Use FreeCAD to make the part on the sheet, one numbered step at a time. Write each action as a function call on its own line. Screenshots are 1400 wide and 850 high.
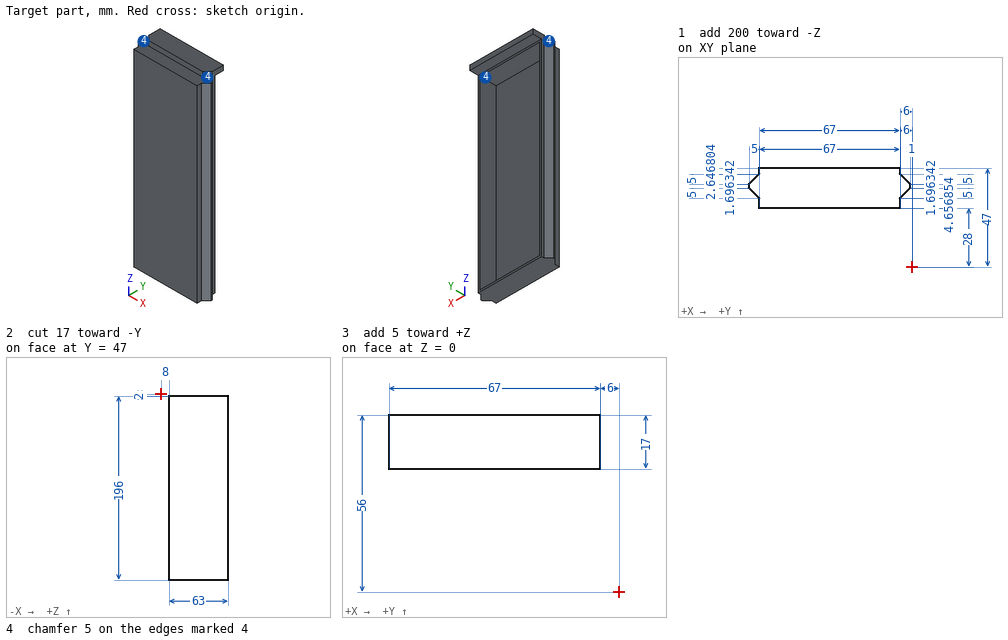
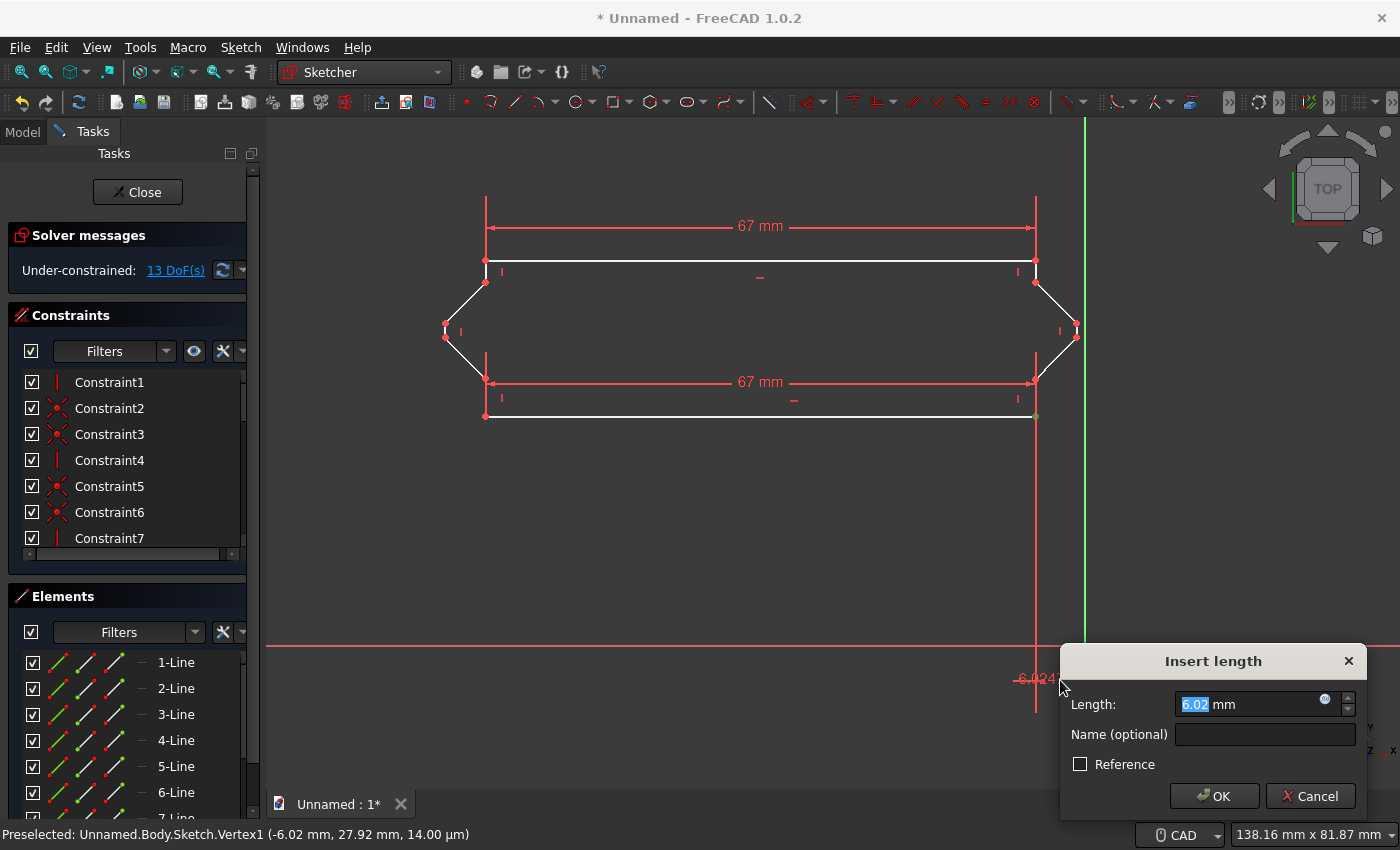
text(6)
key(Return)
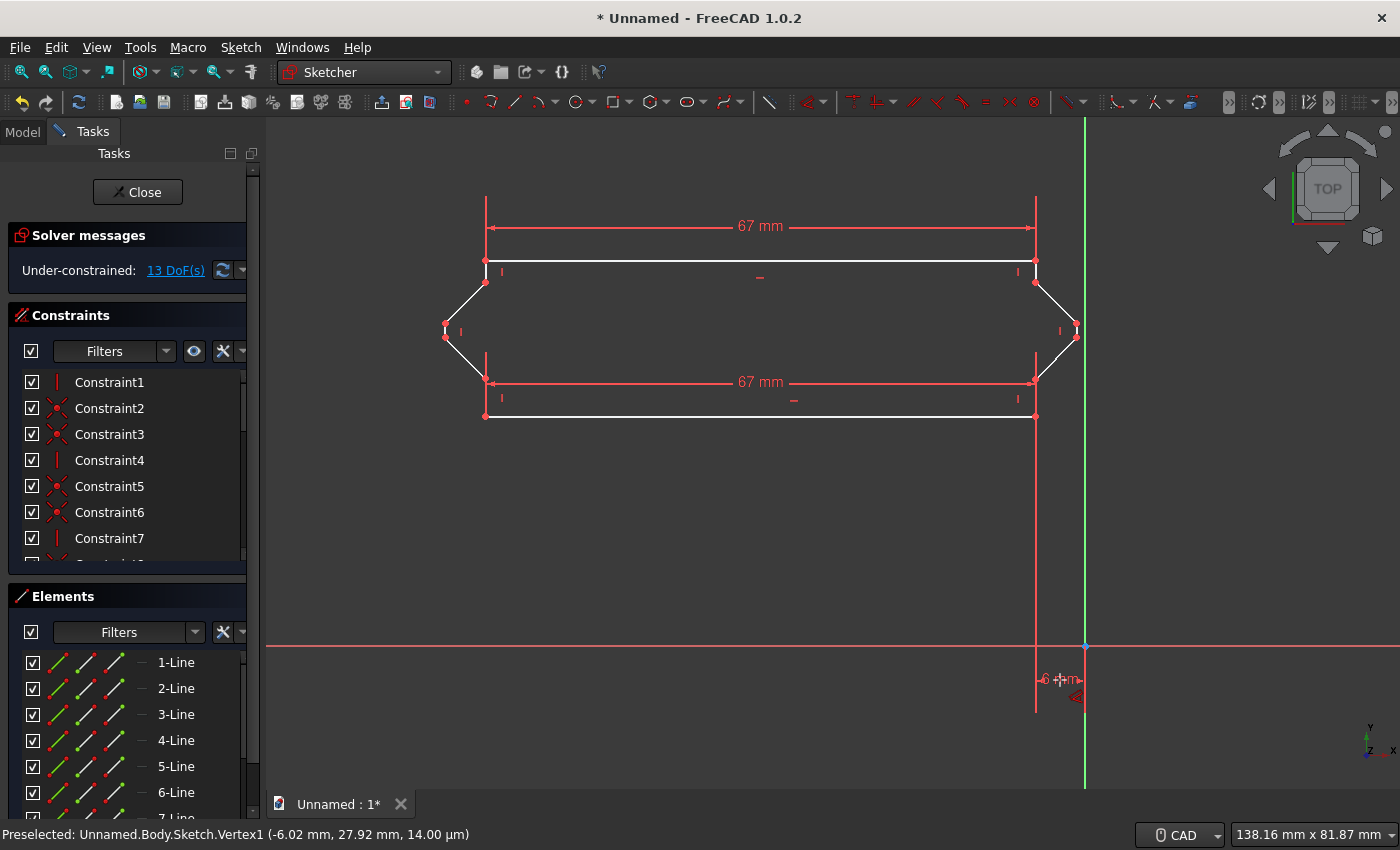
scroll(1077, 338, up, 8)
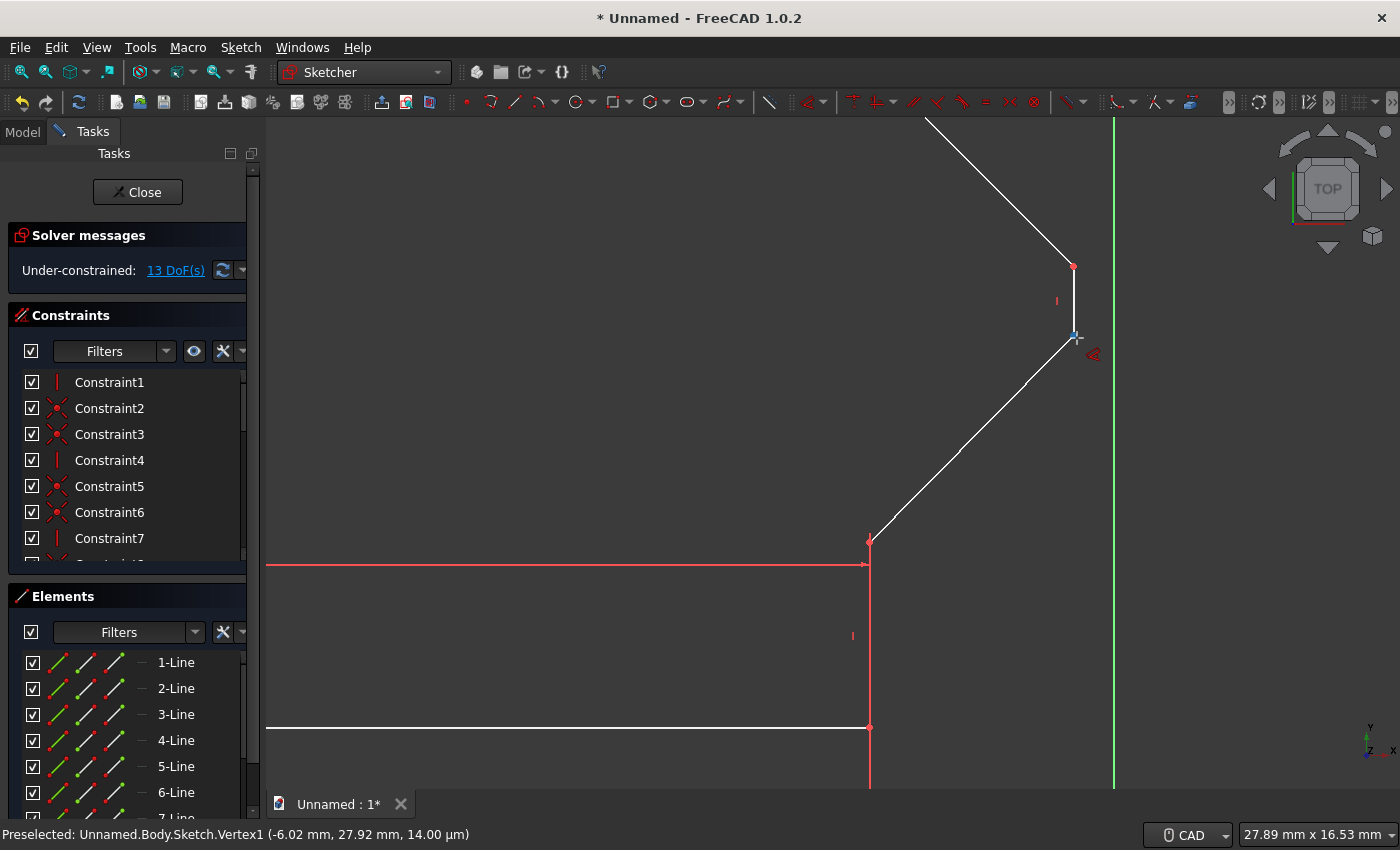
click(1074, 335)
click(1094, 301)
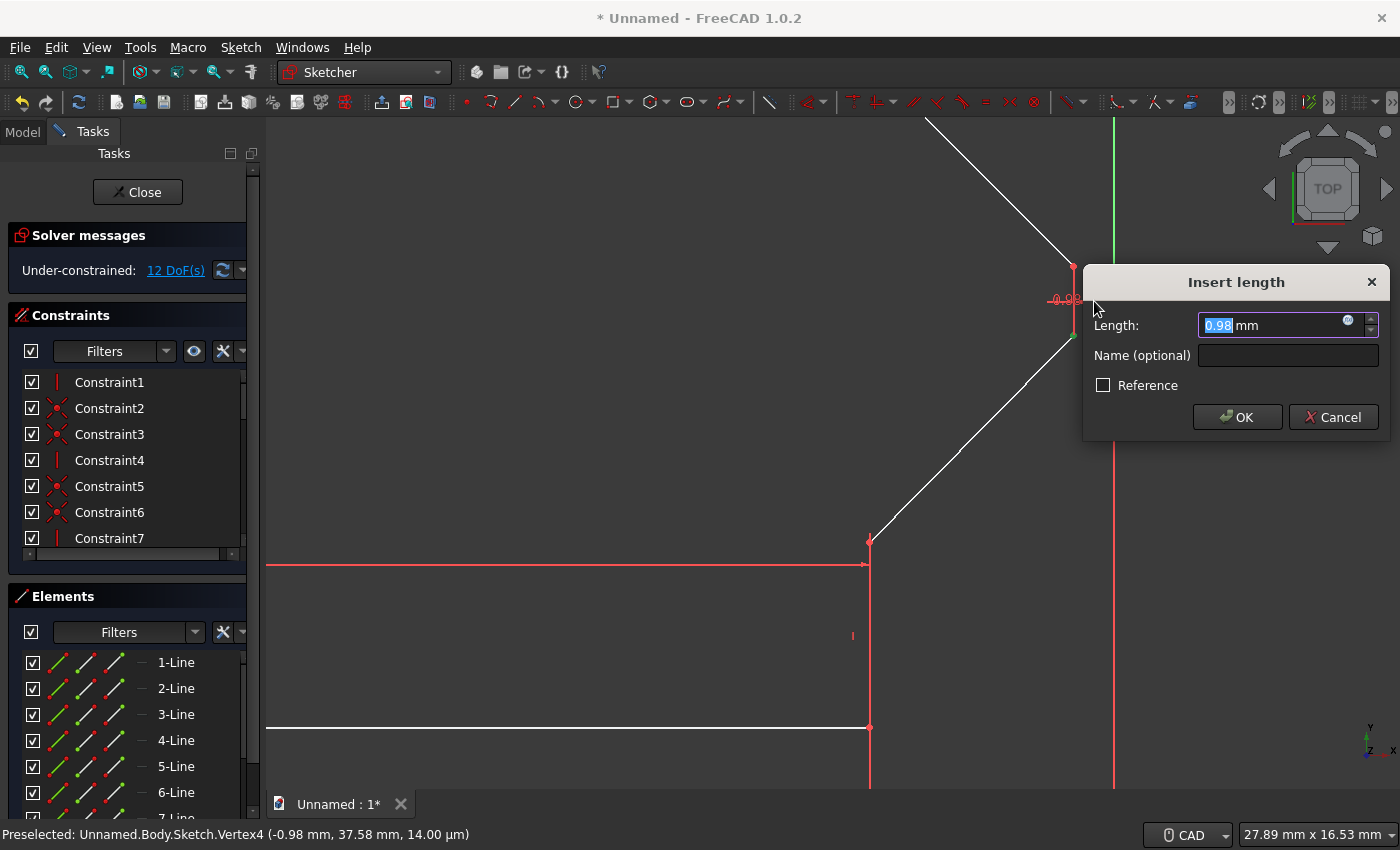
text(1)
key(Return)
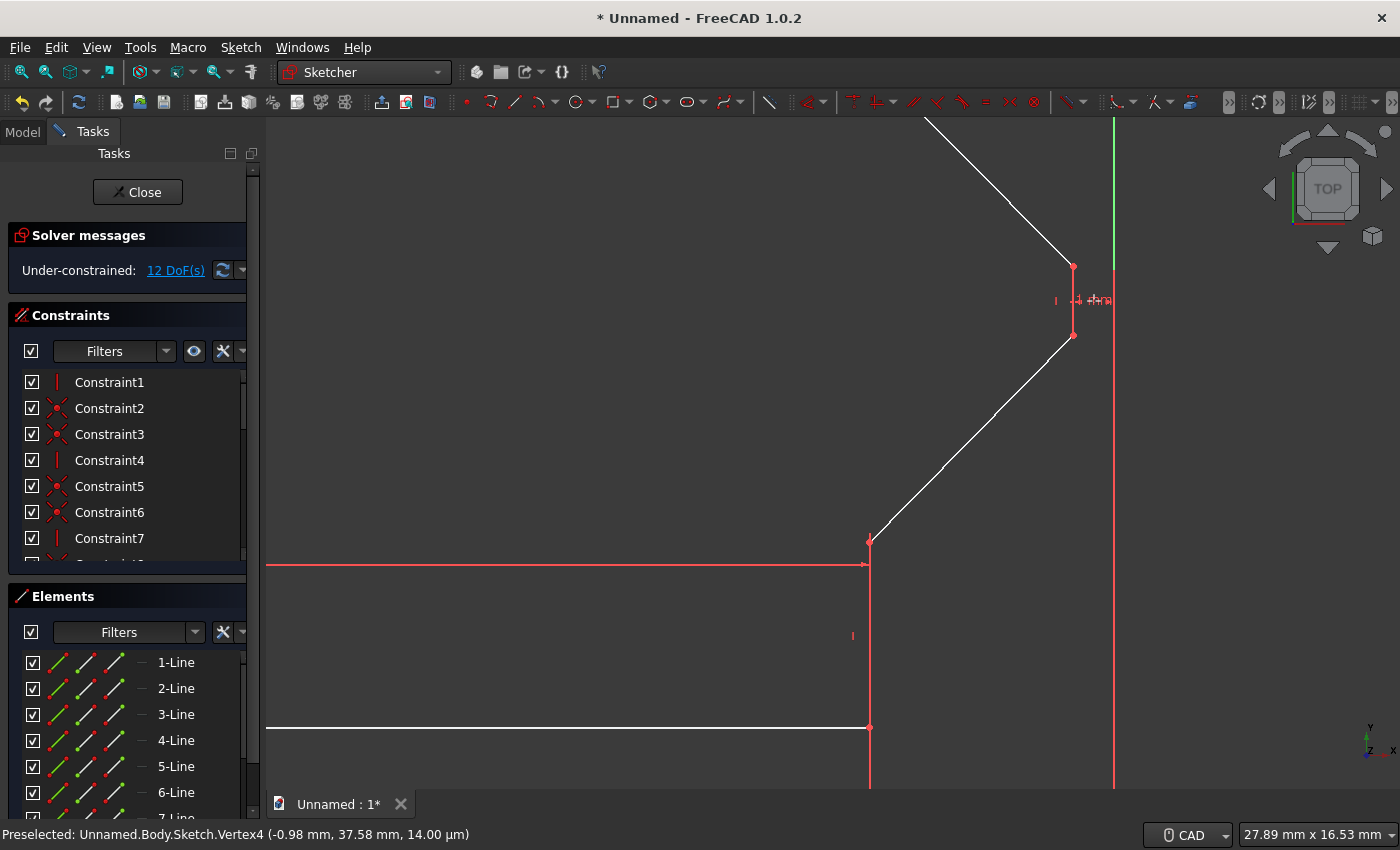
scroll(1077, 338, down, 8)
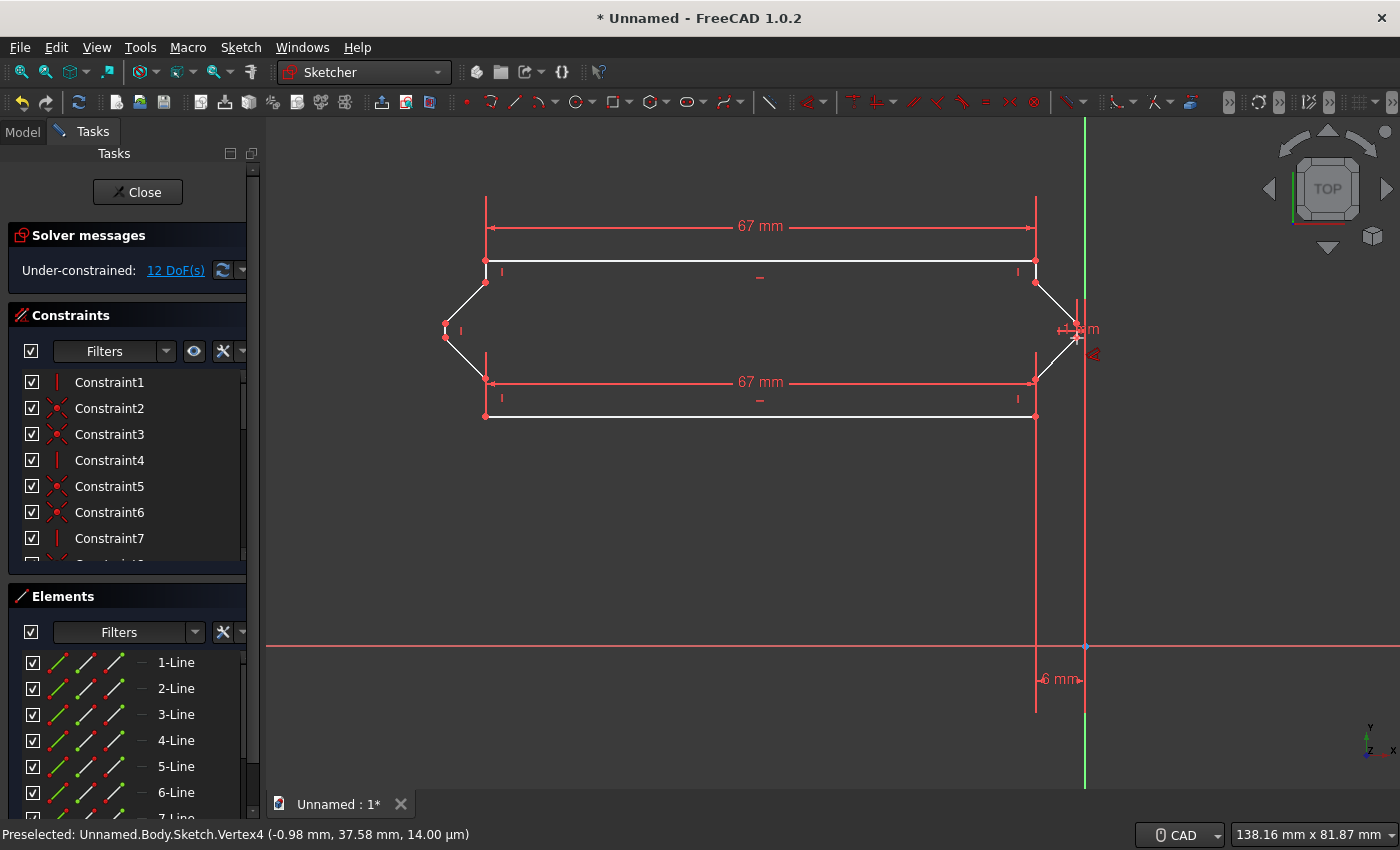
click(1036, 282)
click(1060, 248)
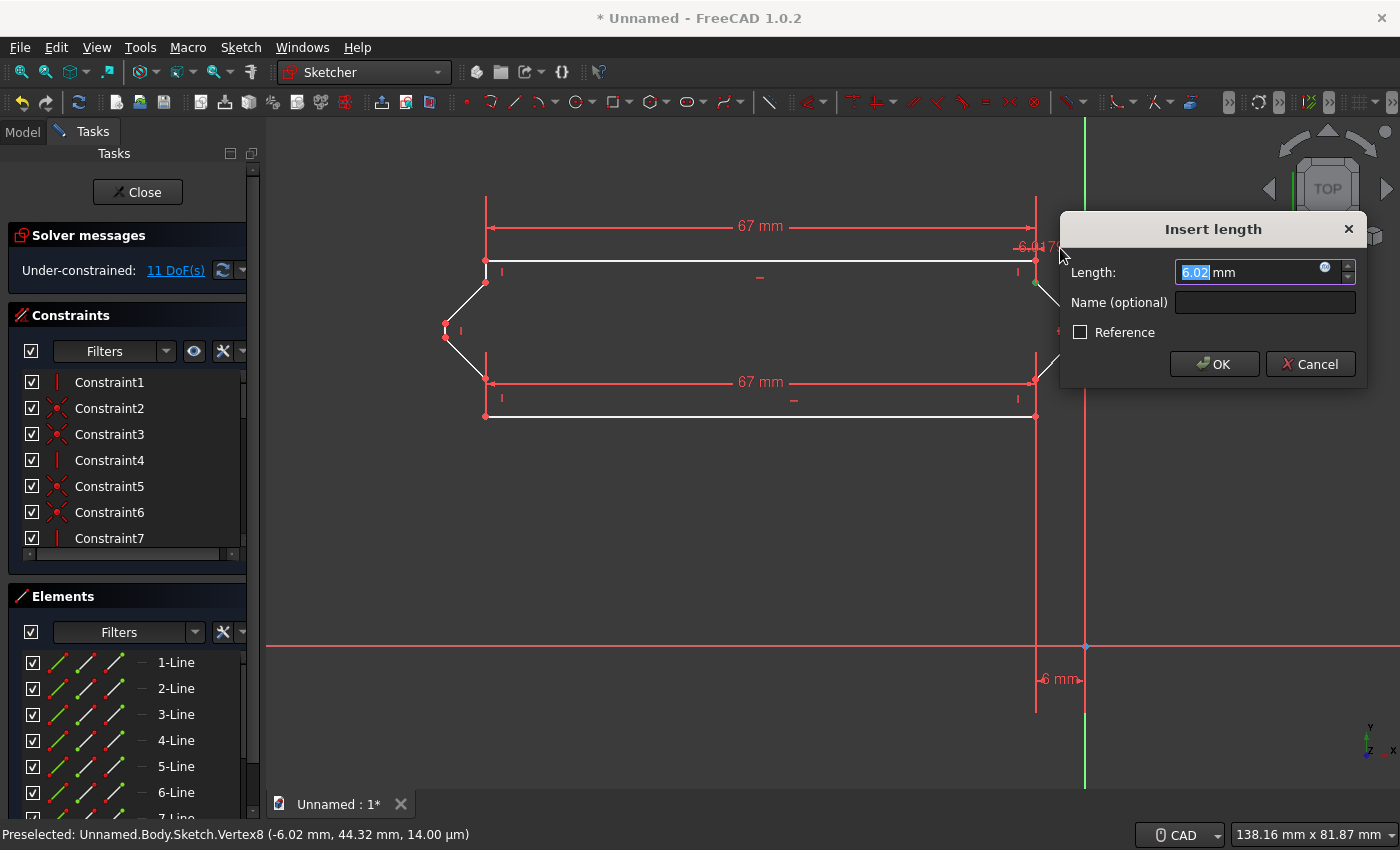
text(6)
key(Return)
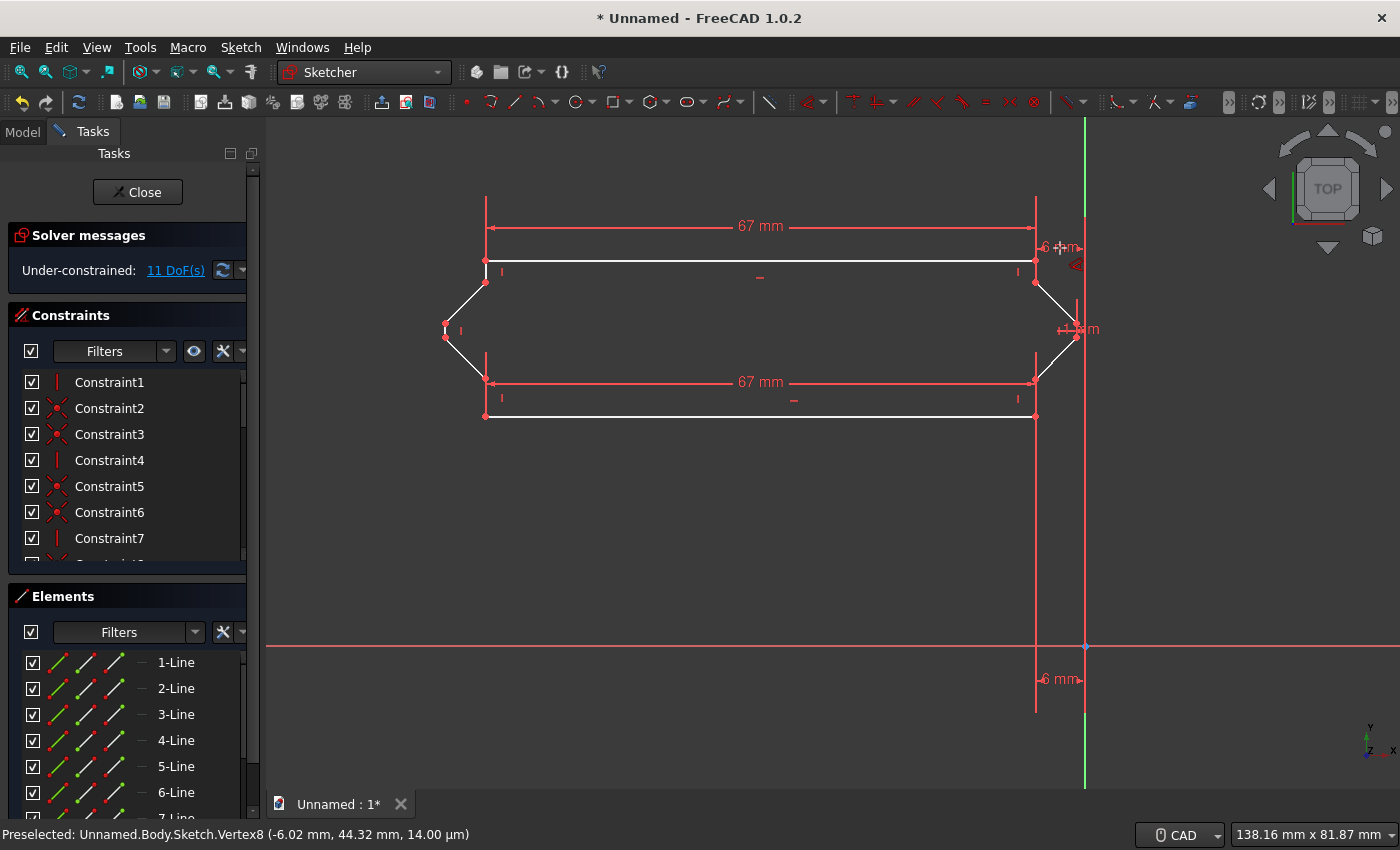
click(1048, 367)
click(1111, 359)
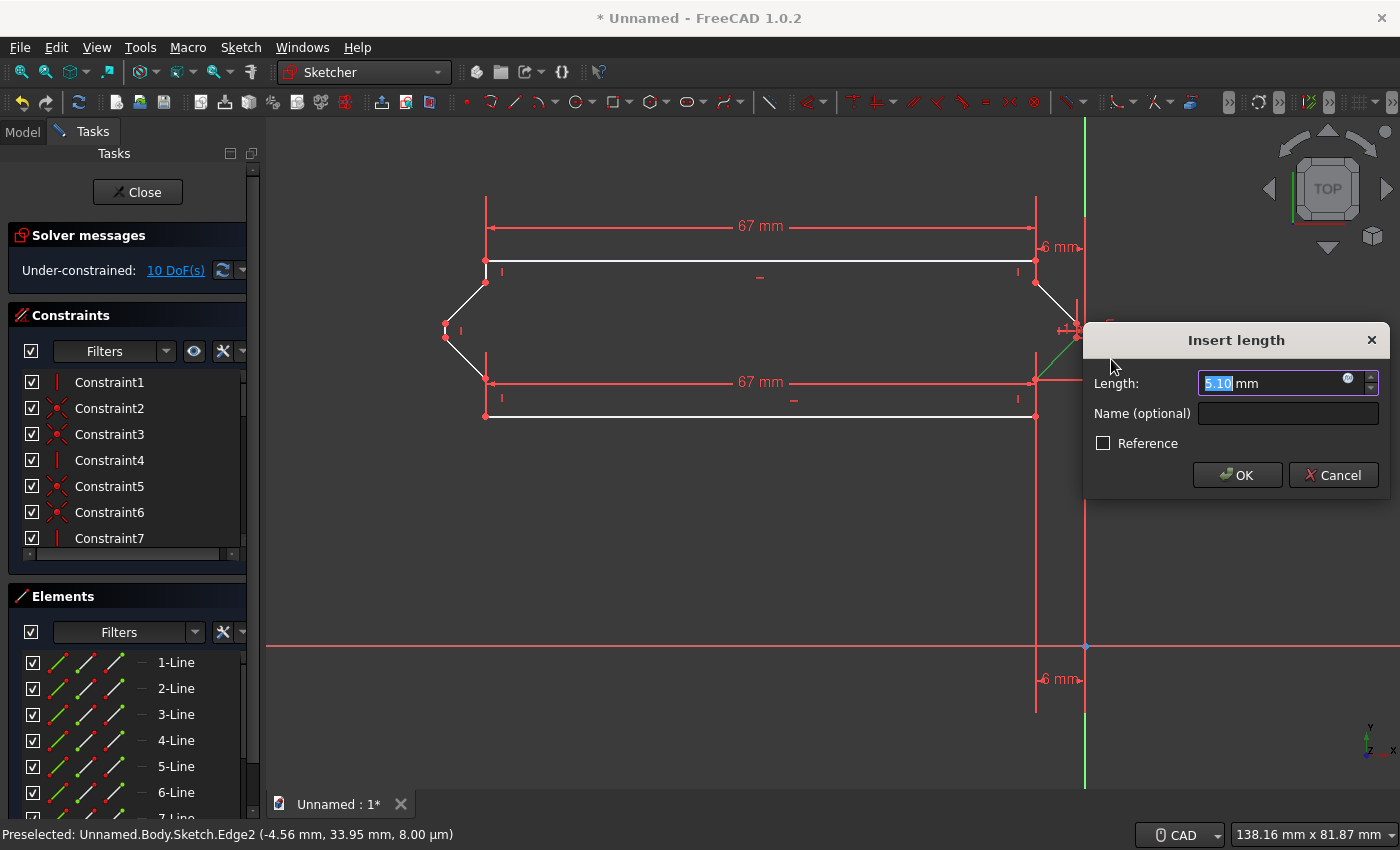
text(5)
key(Return)